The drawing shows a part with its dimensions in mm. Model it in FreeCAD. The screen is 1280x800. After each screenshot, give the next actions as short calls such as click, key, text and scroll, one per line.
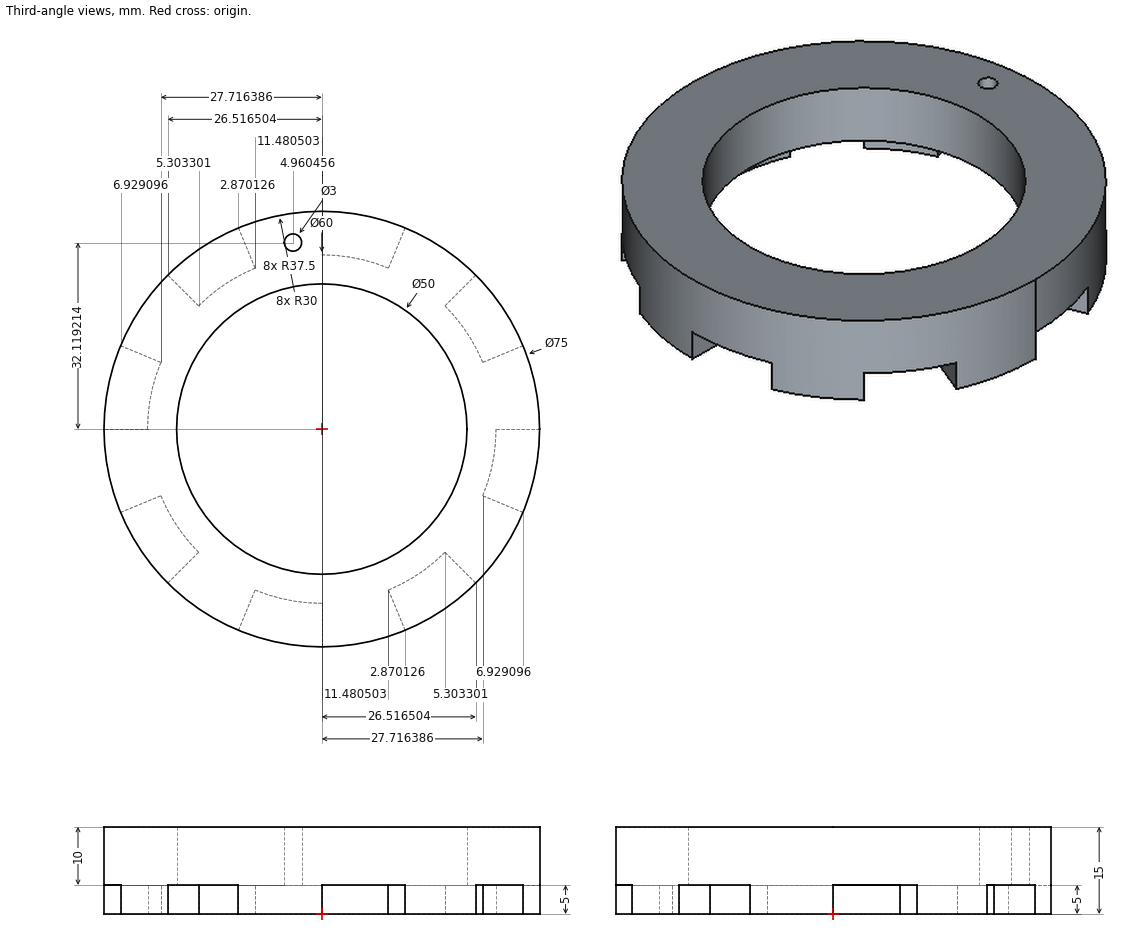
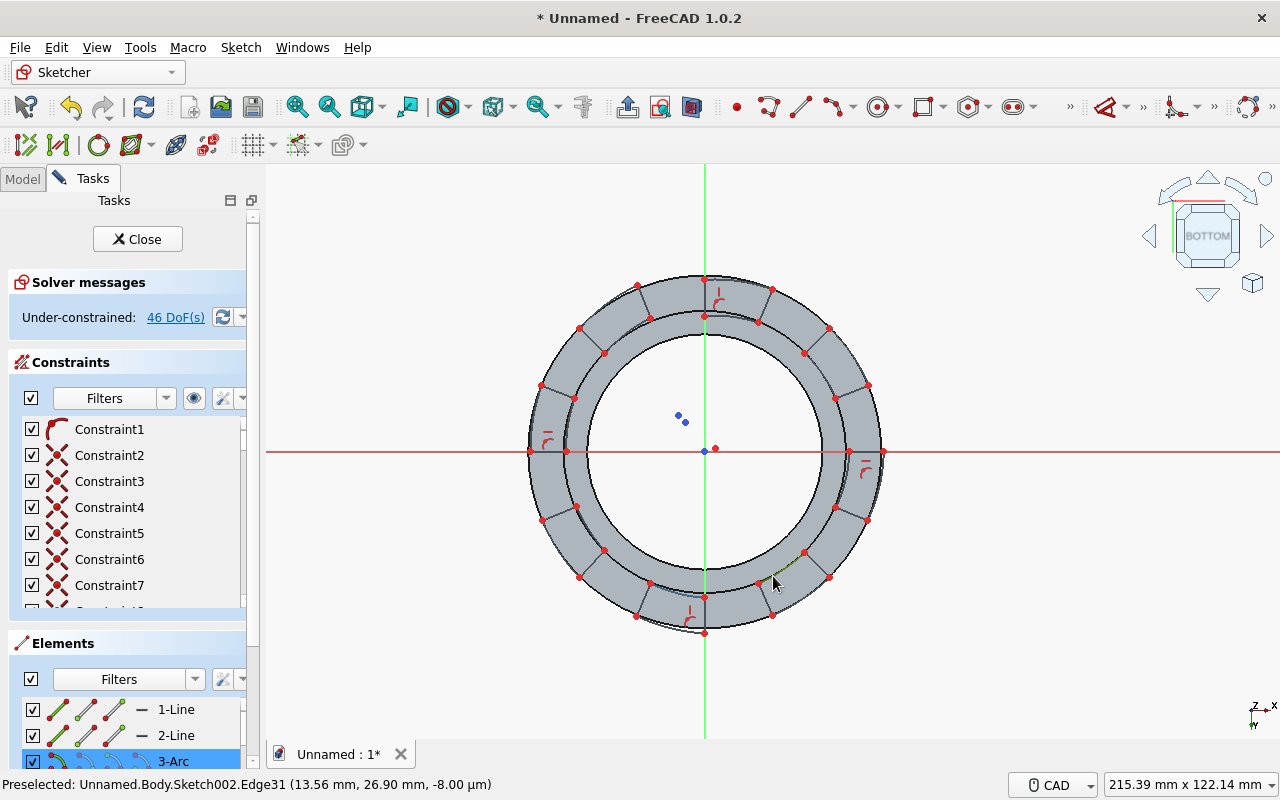
key(c)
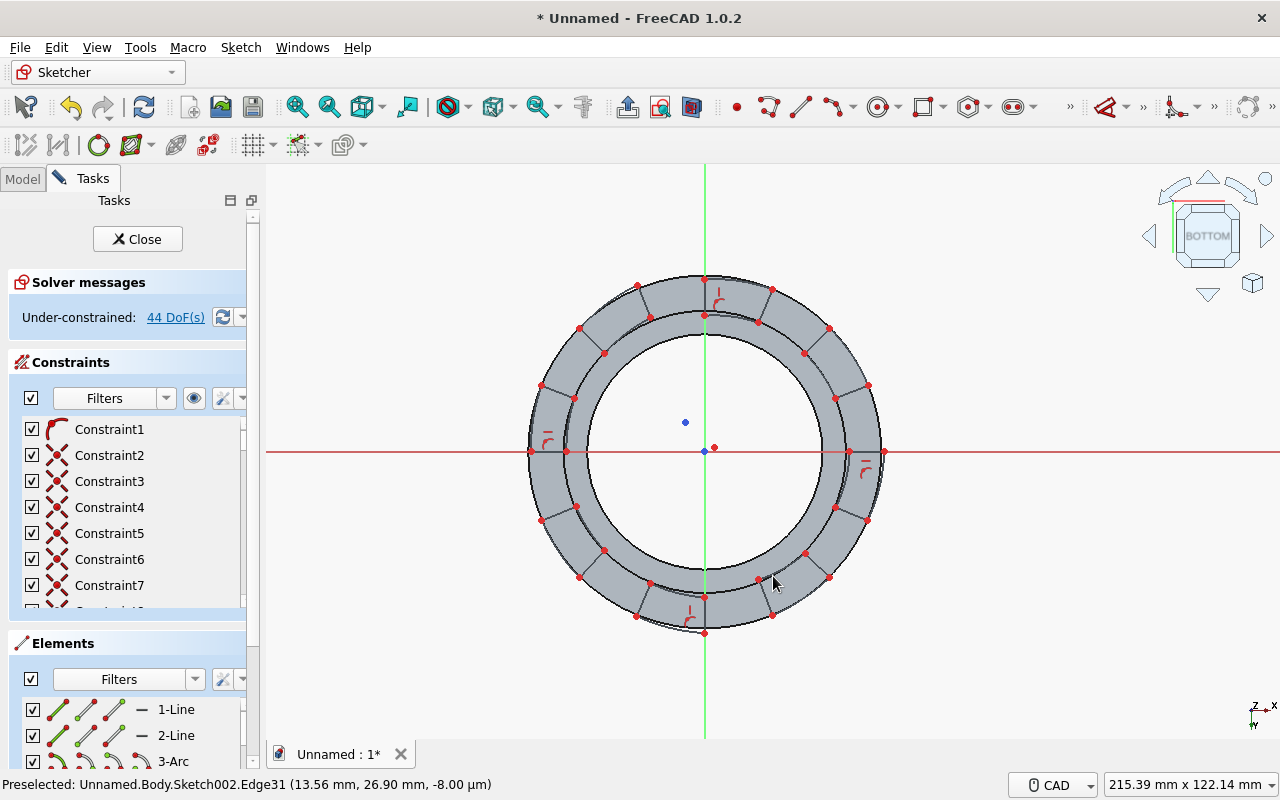
click(666, 590)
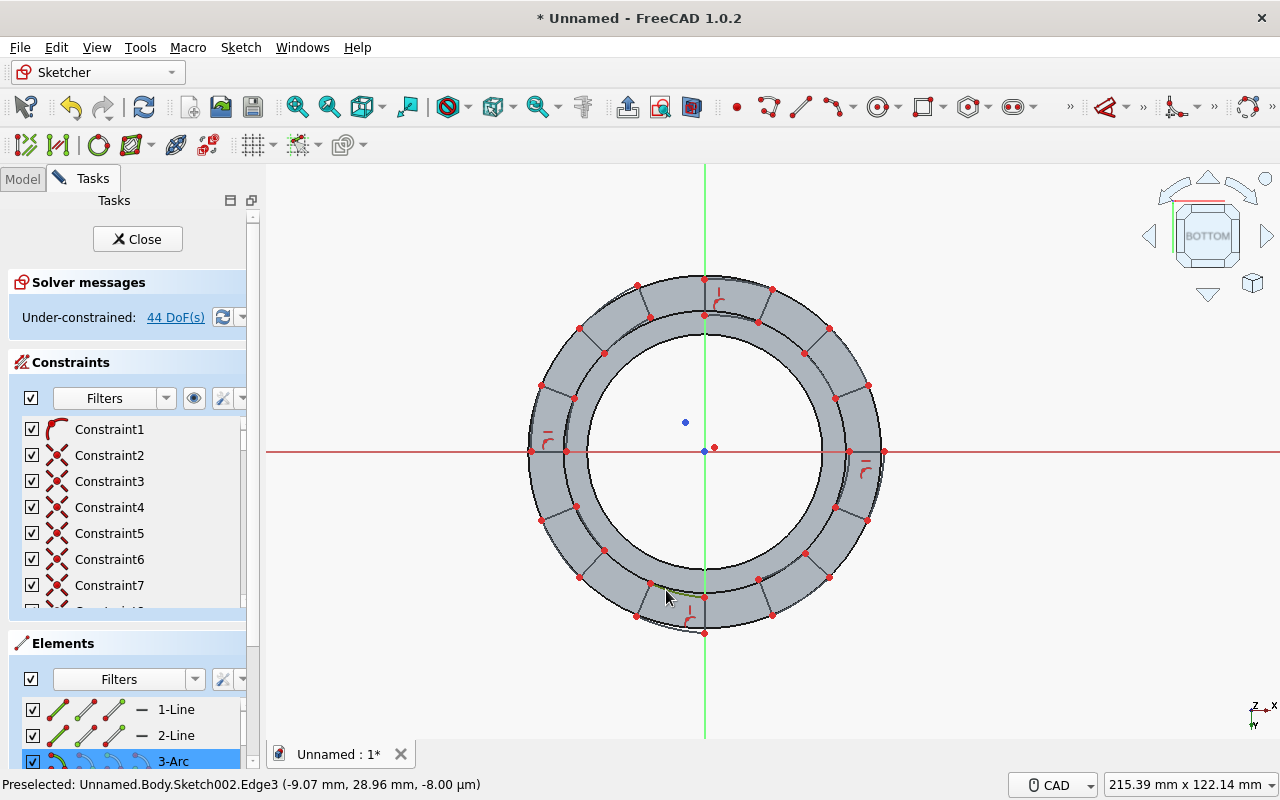
click(791, 606)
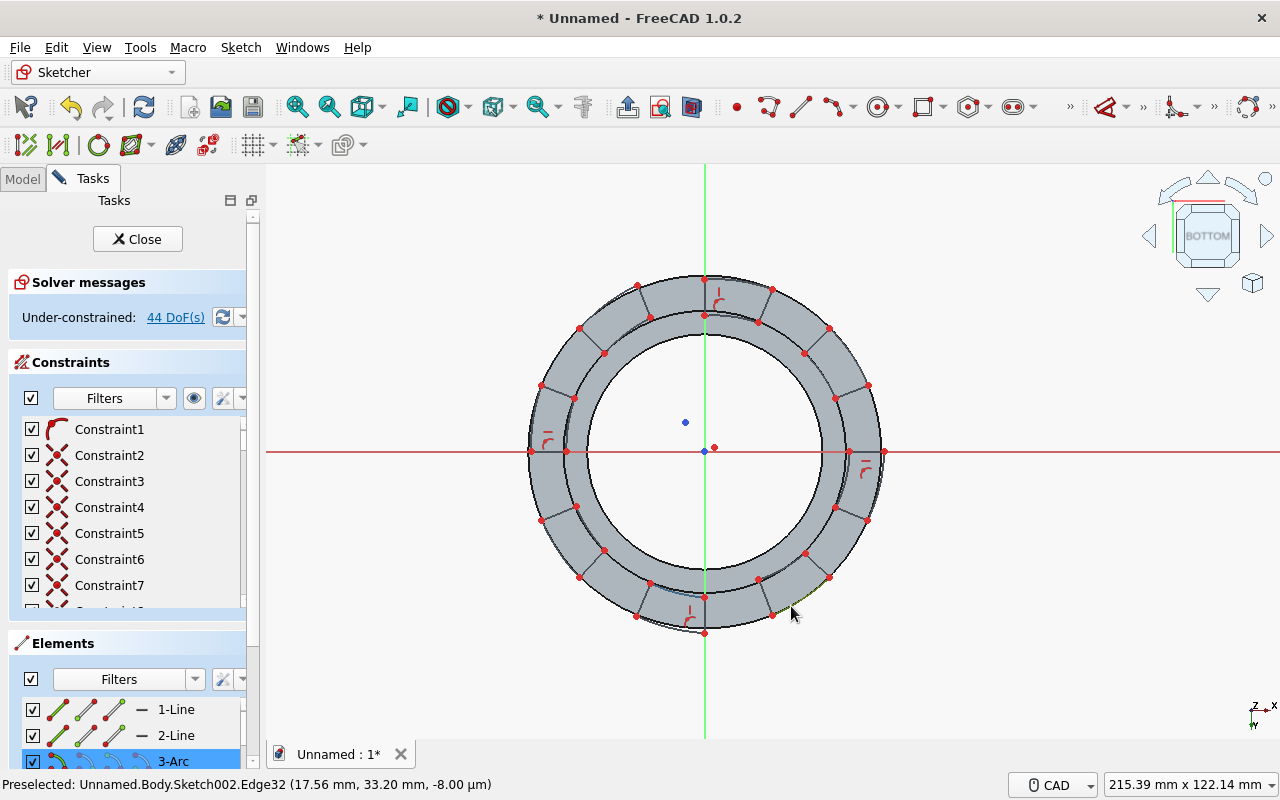
key(c)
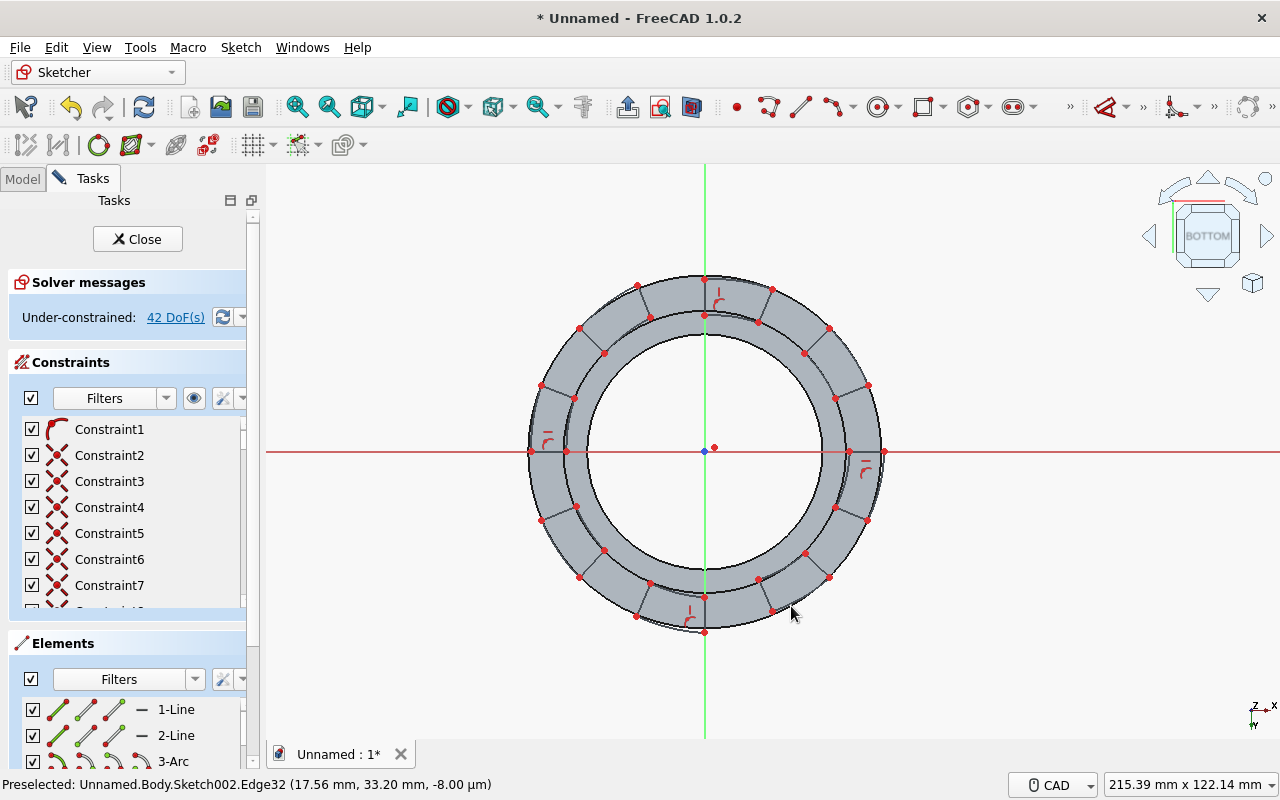
drag(695, 437, 724, 462)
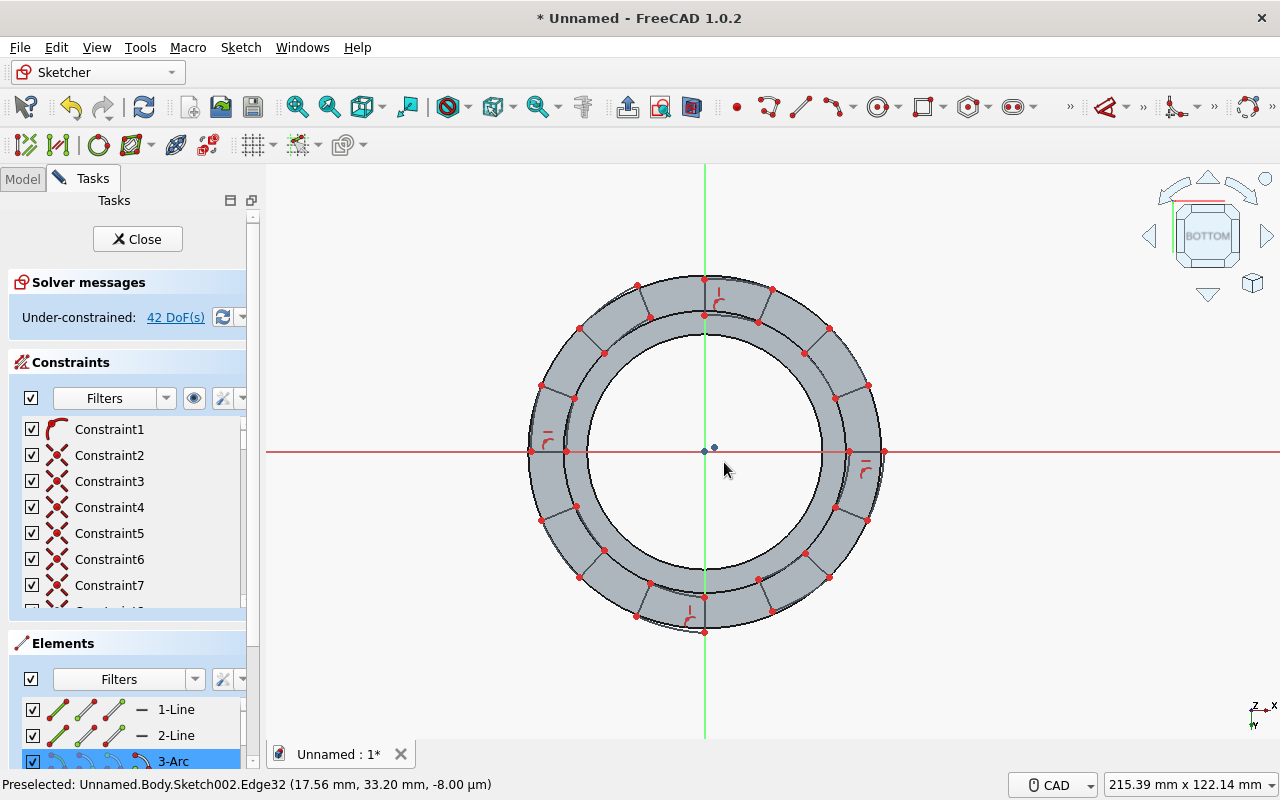
key(c)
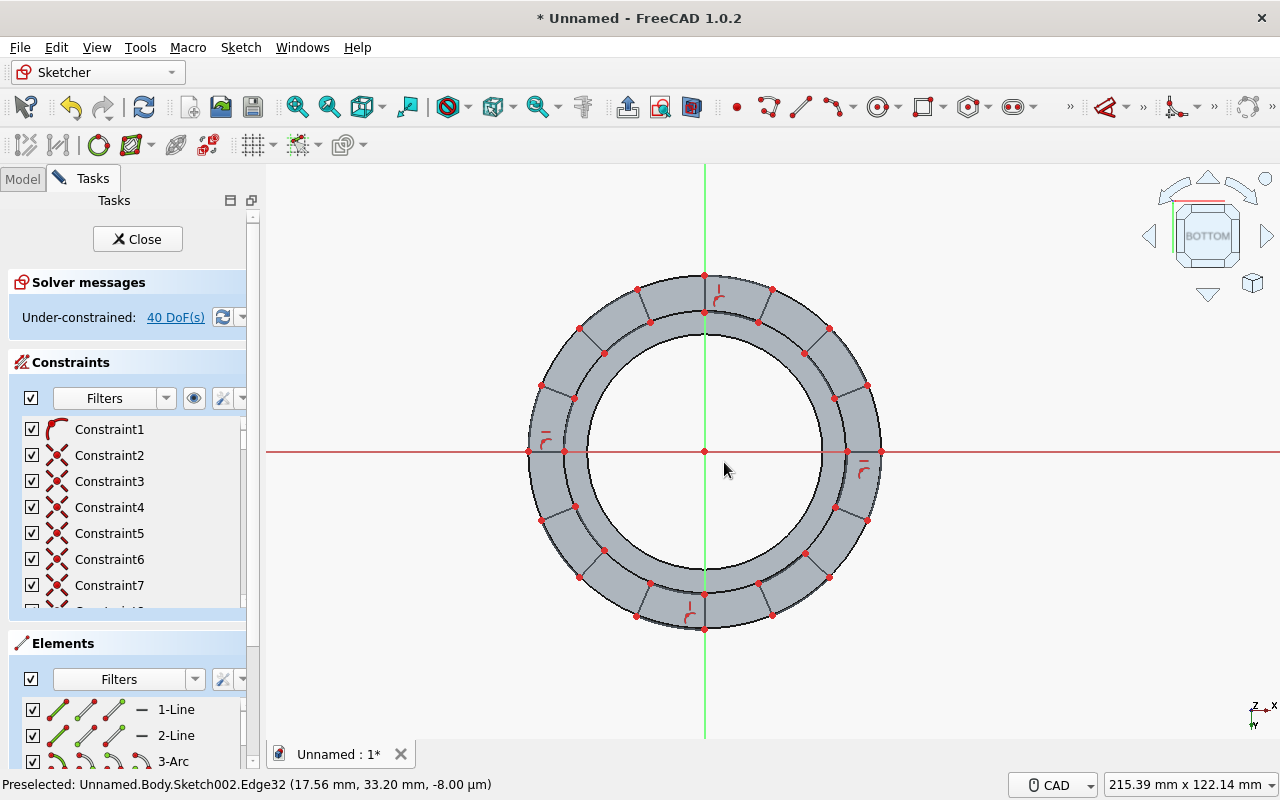
click(666, 589)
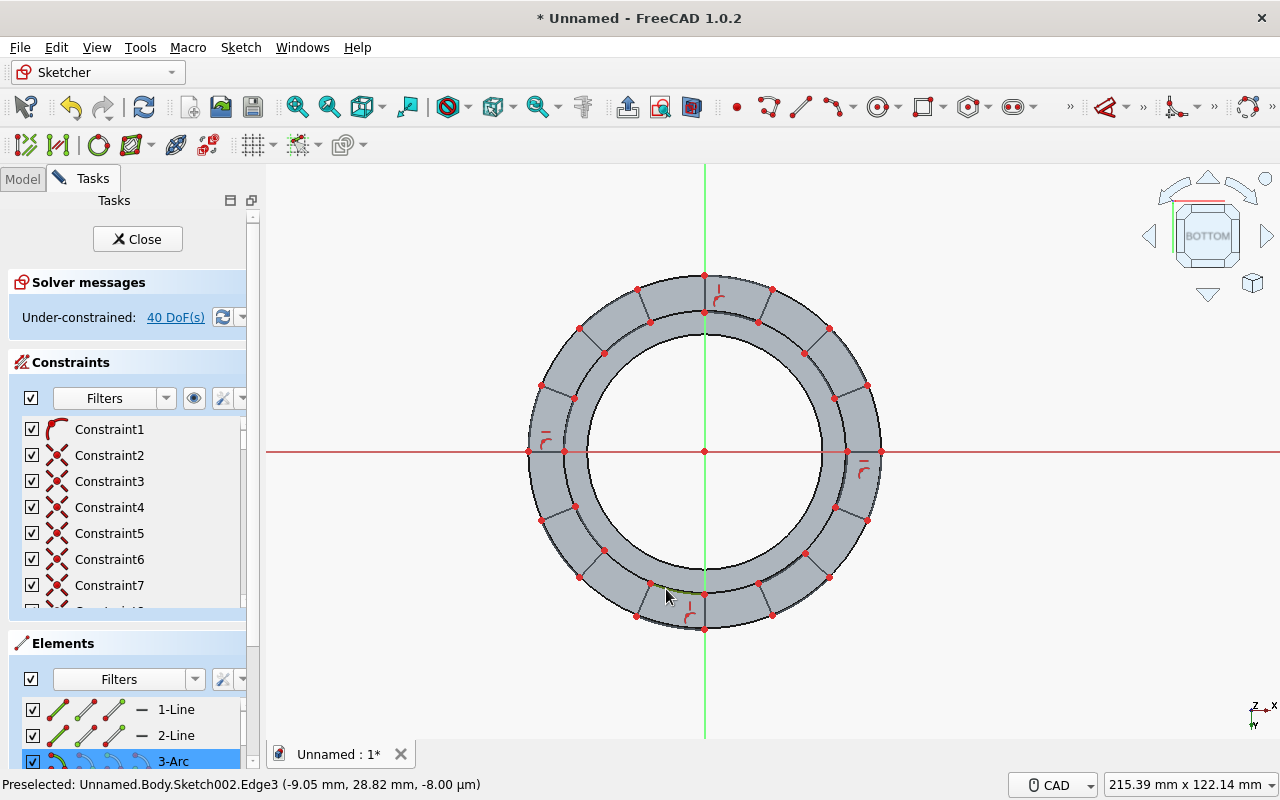
click(582, 521)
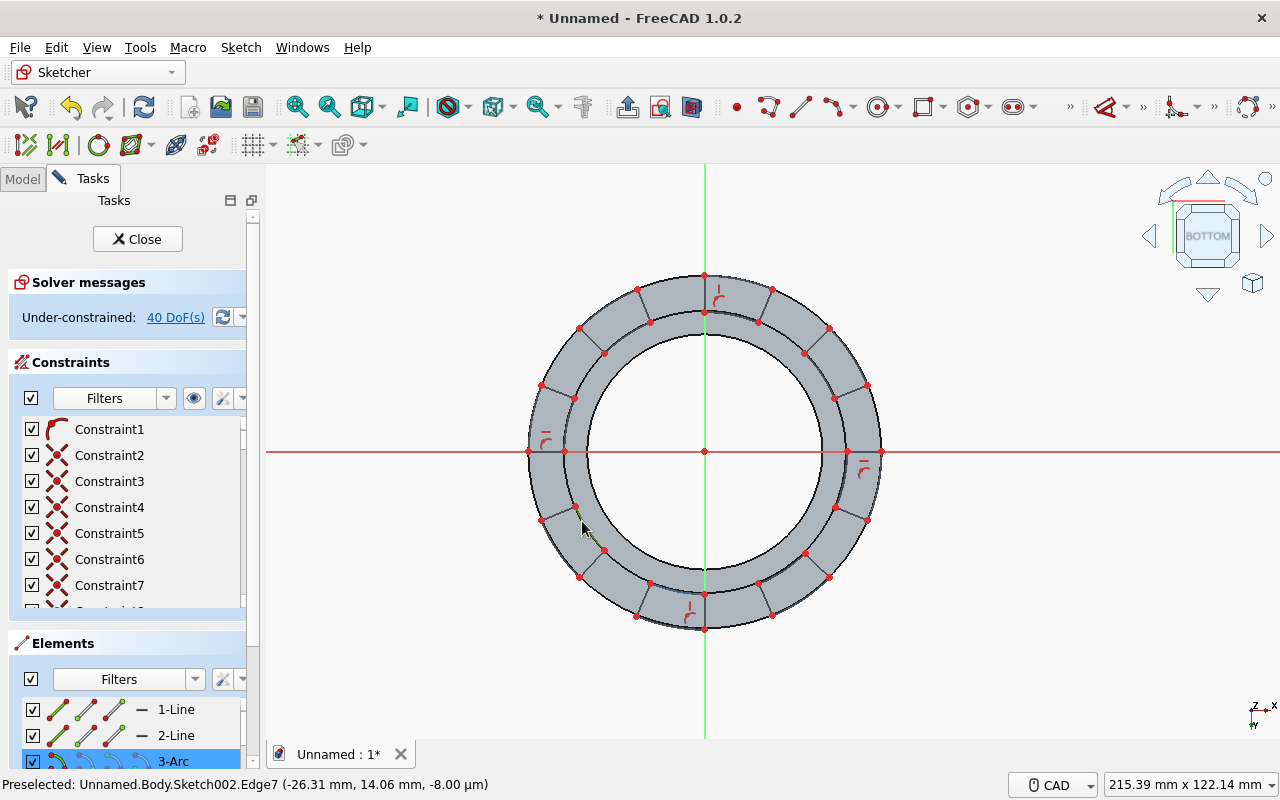
click(569, 414)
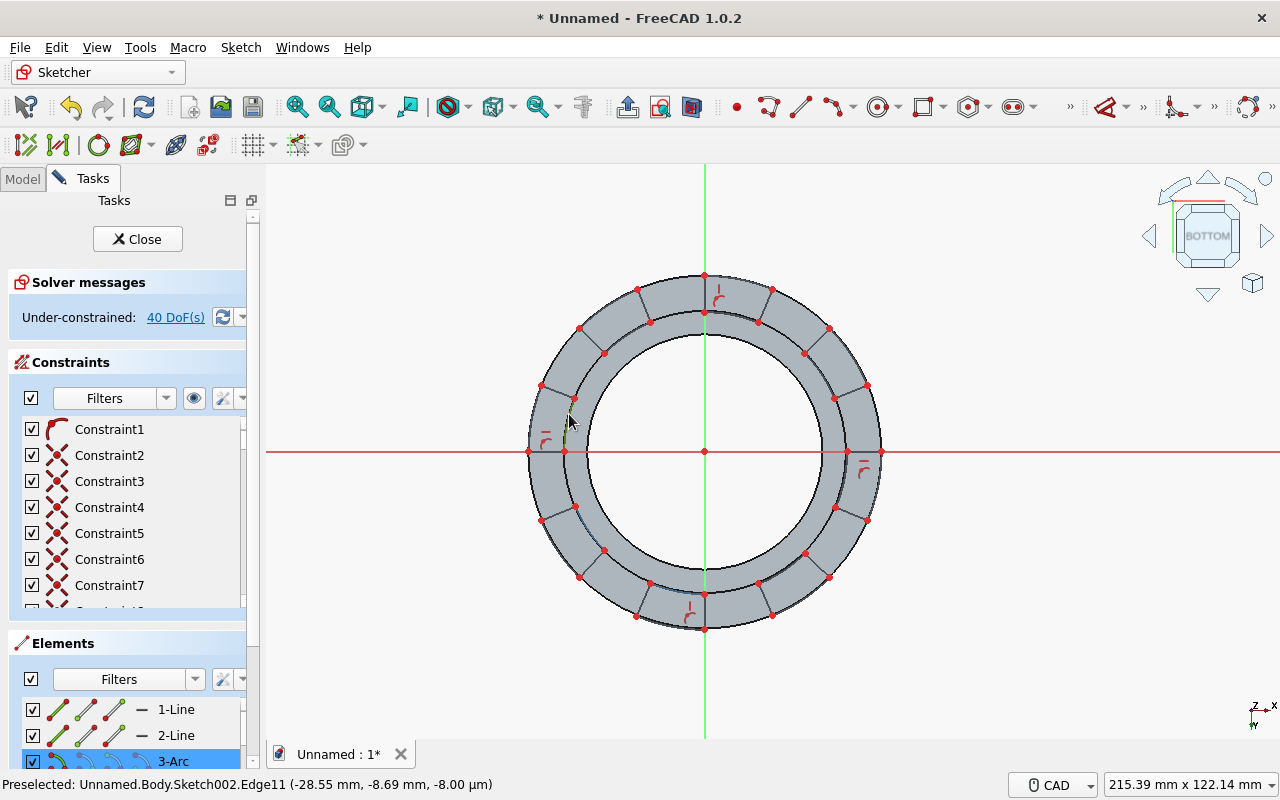
click(636, 330)